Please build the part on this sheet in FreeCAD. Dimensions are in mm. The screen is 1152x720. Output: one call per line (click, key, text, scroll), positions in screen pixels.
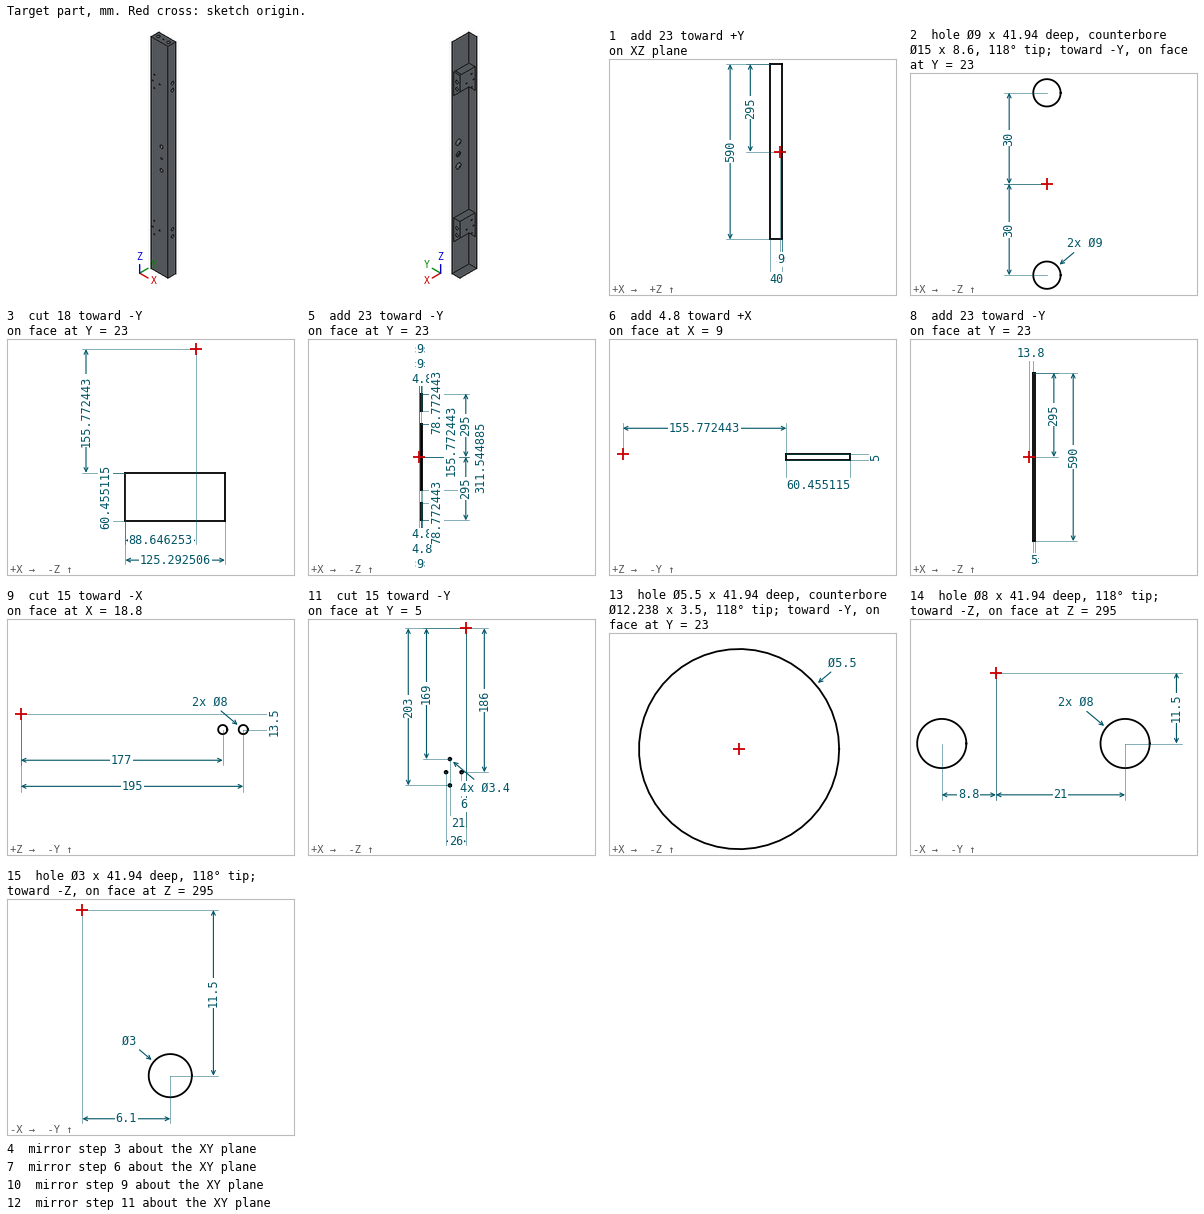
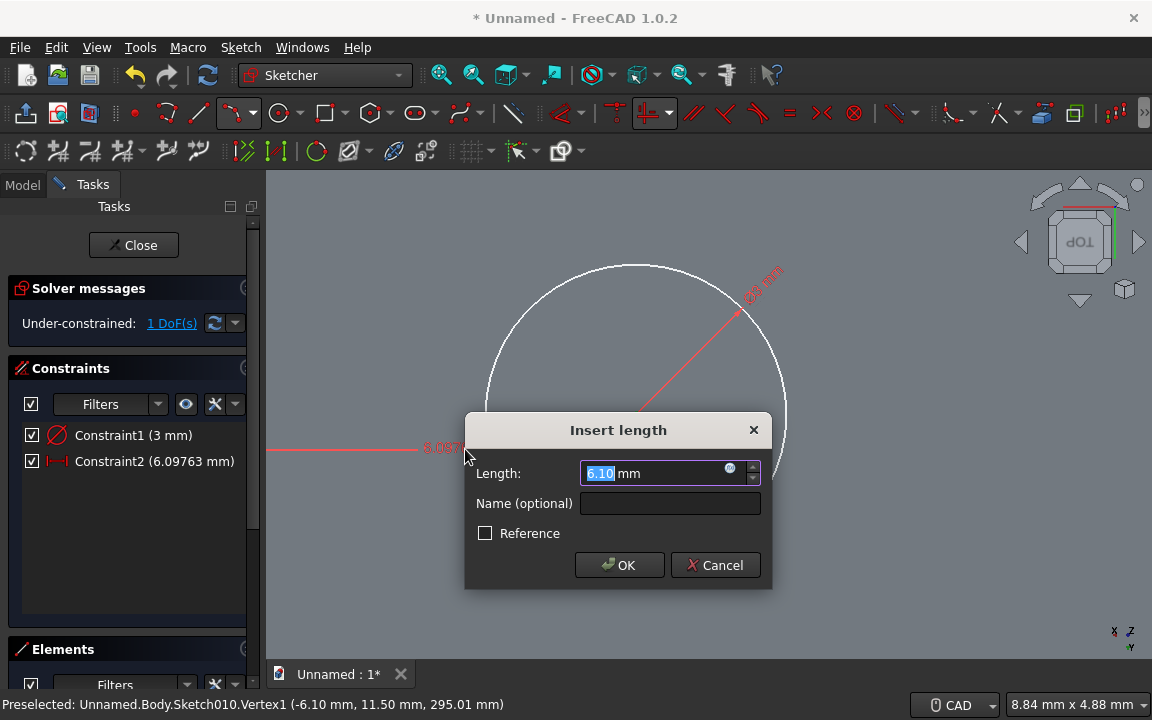
text(6.1)
key(Return)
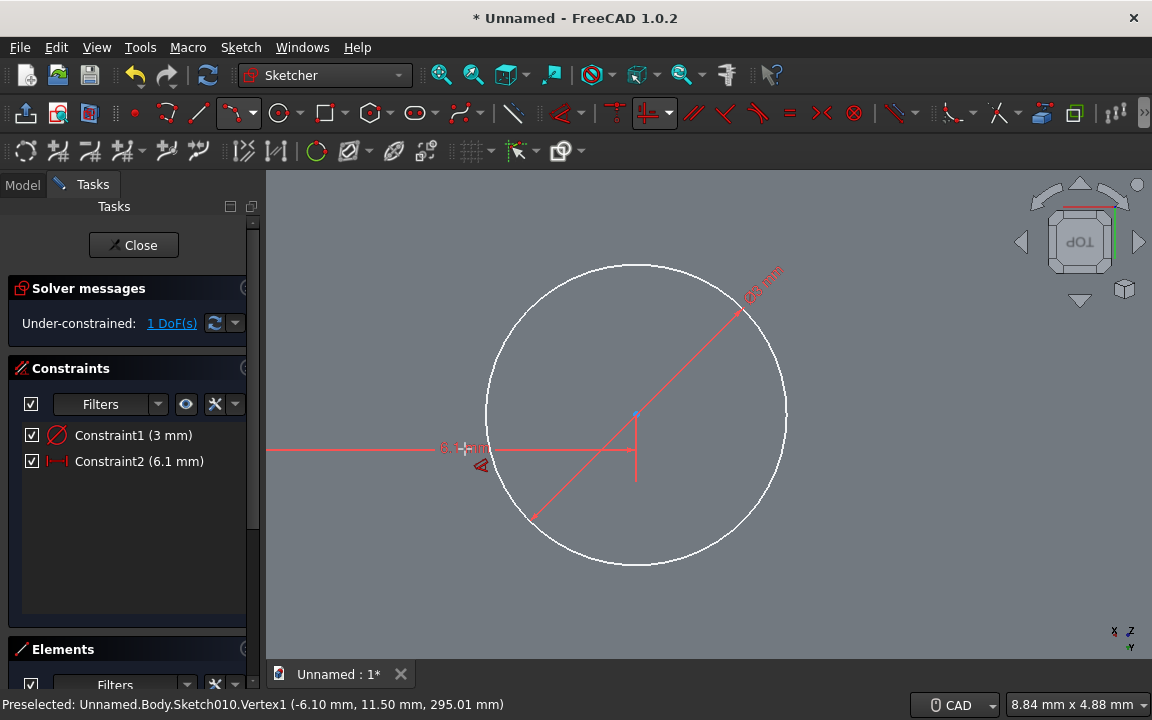
click(636, 415)
click(670, 306)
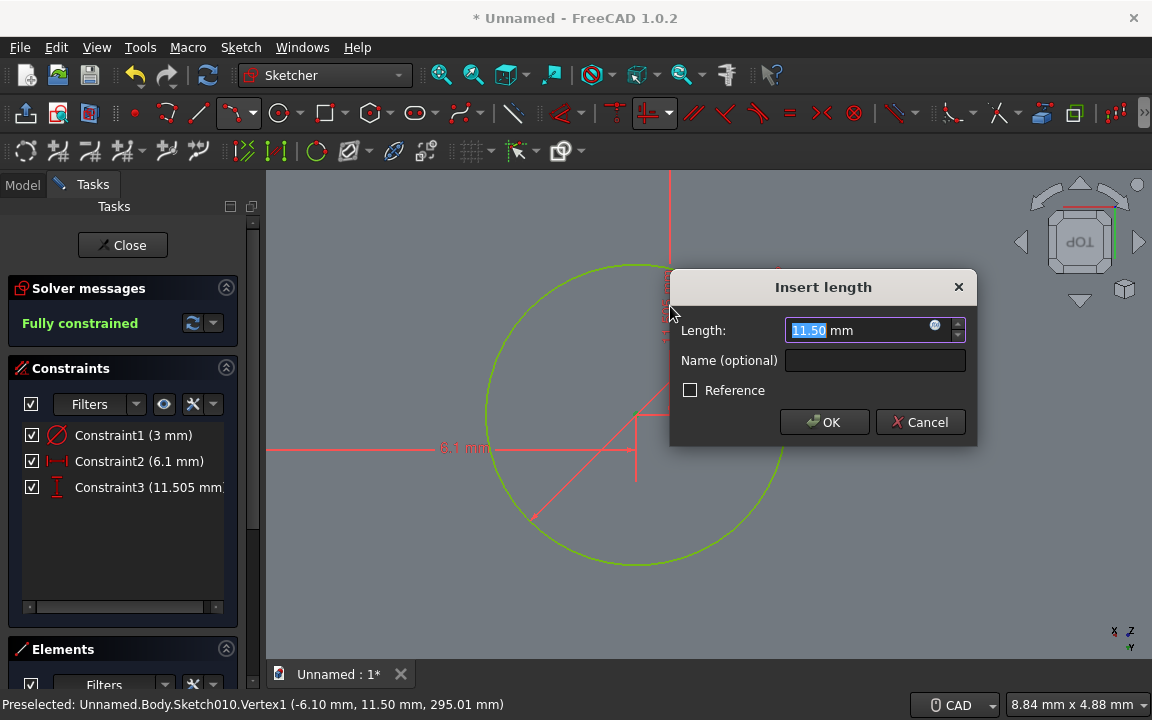
text(11.5)
key(Return)
key(Escape)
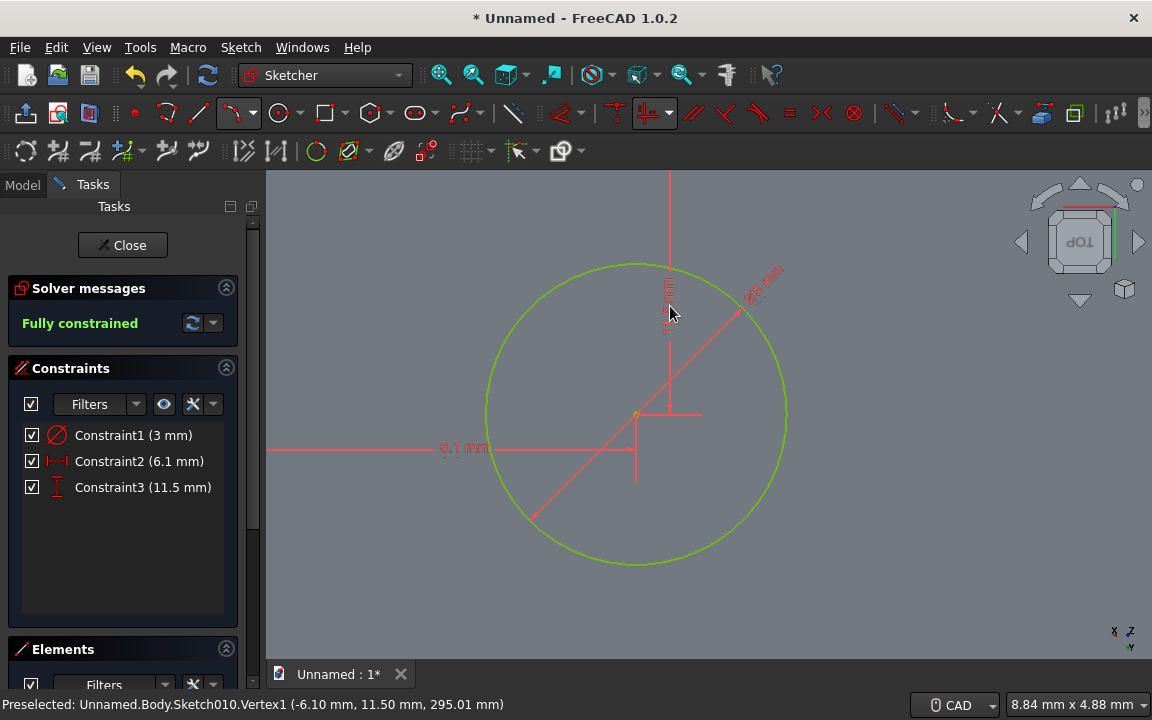
click(123, 245)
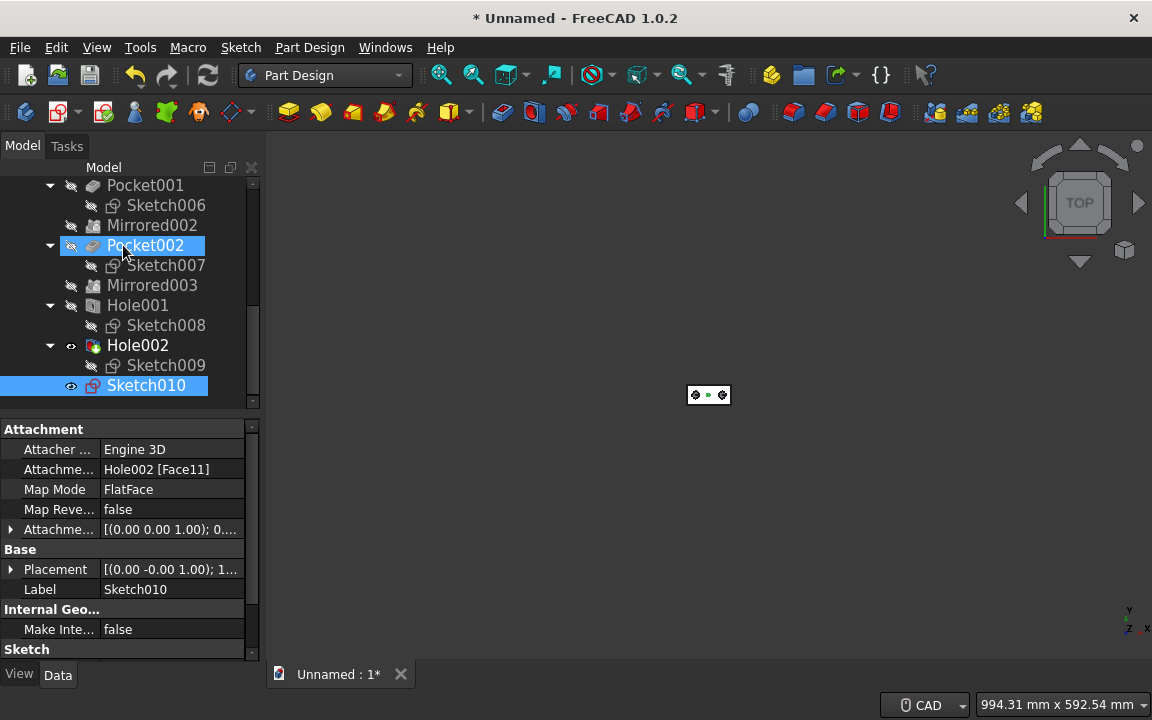
click(536, 112)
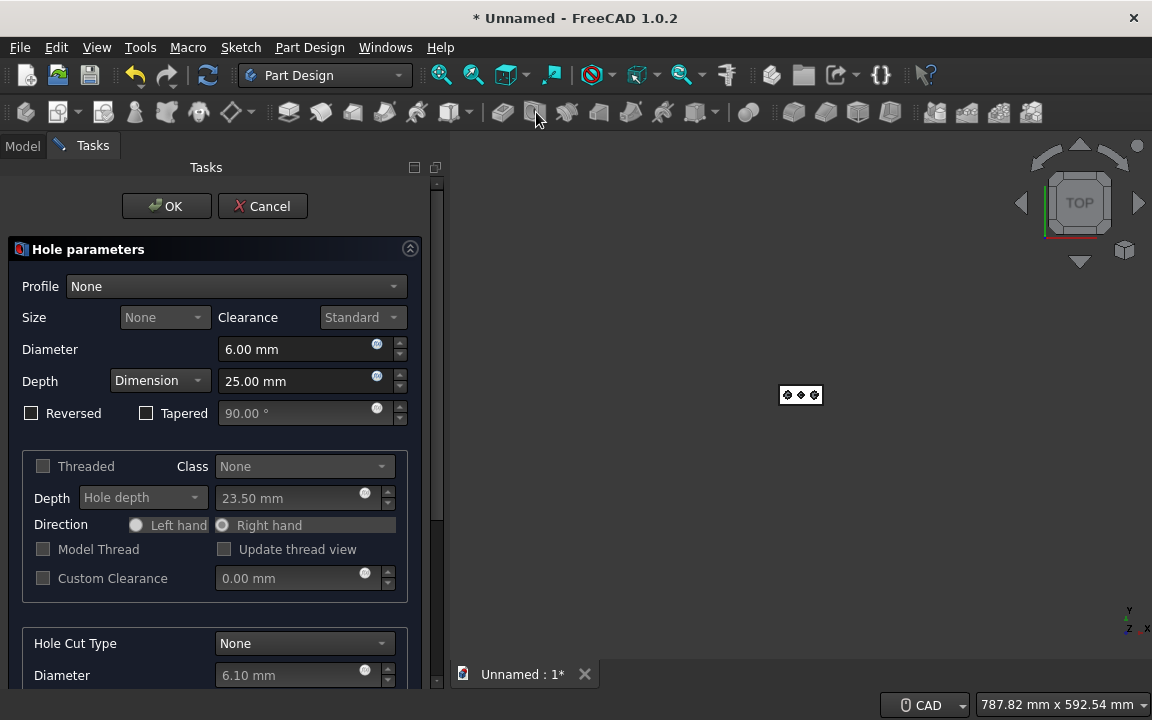
triple_click(305, 349)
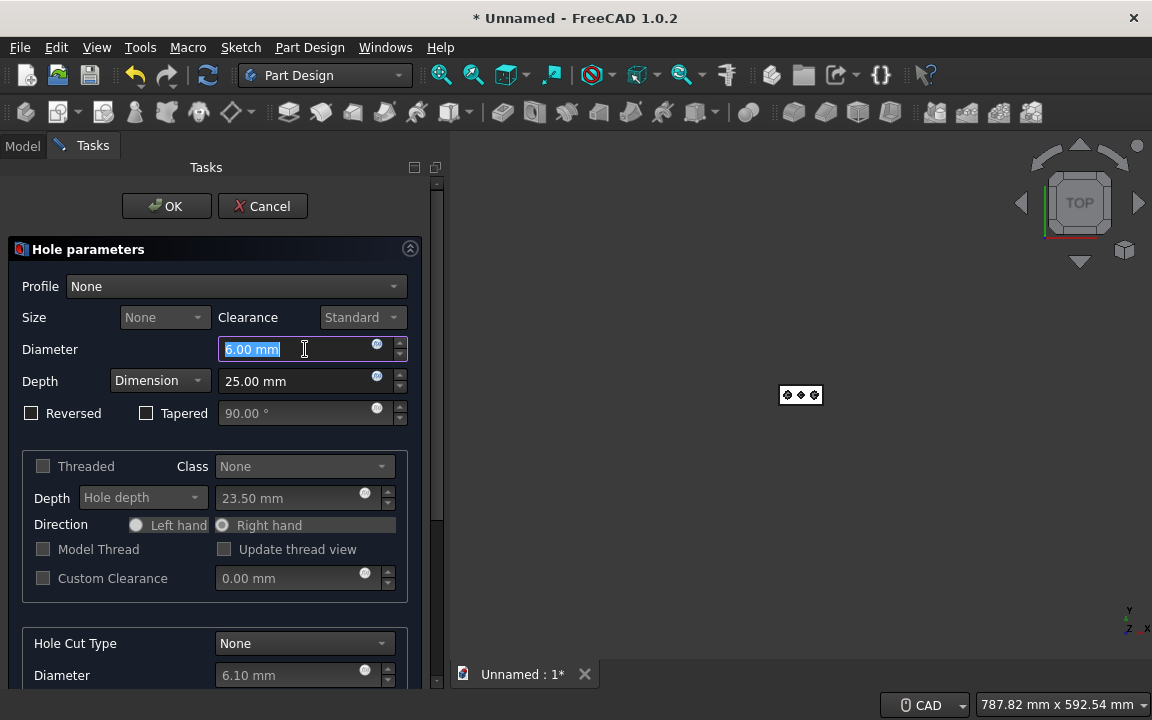
text(3)
key(Tab)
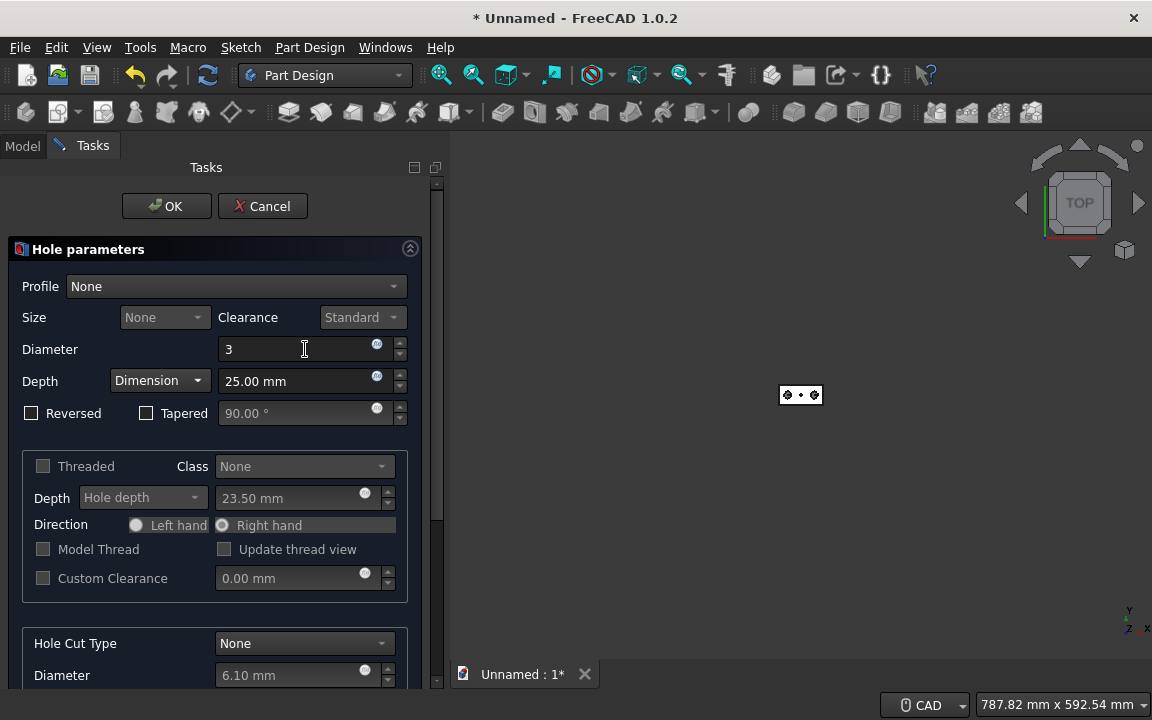
triple_click(305, 381)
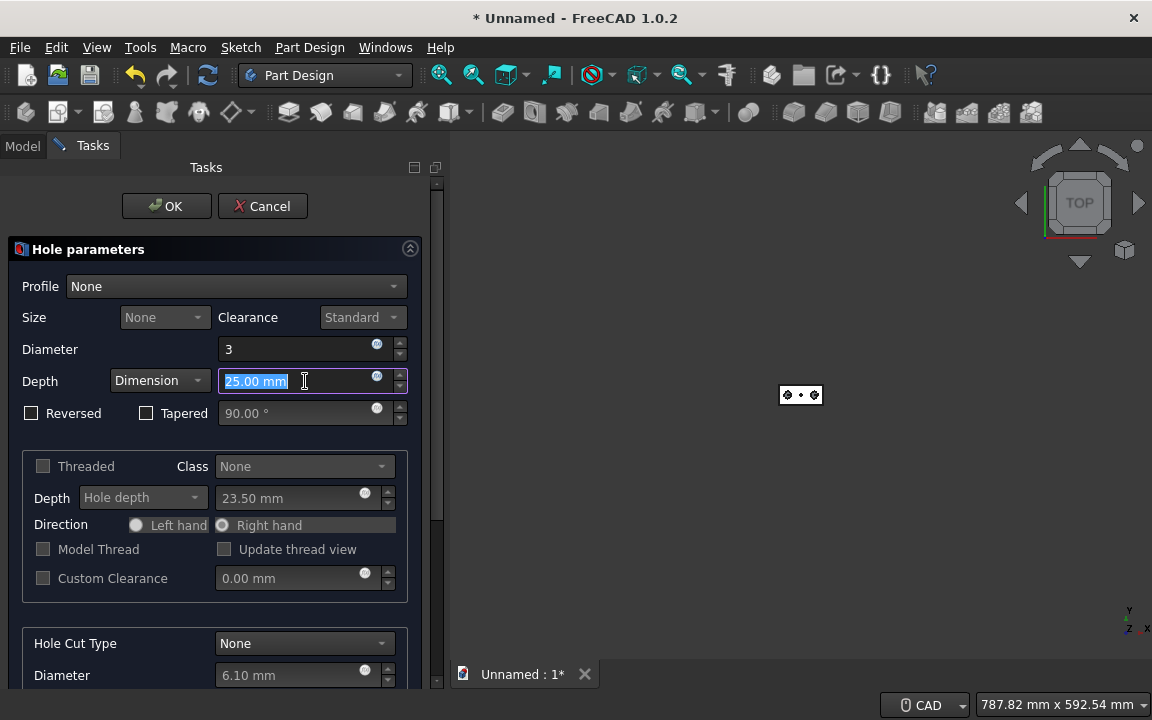
text(41.94)
key(Tab)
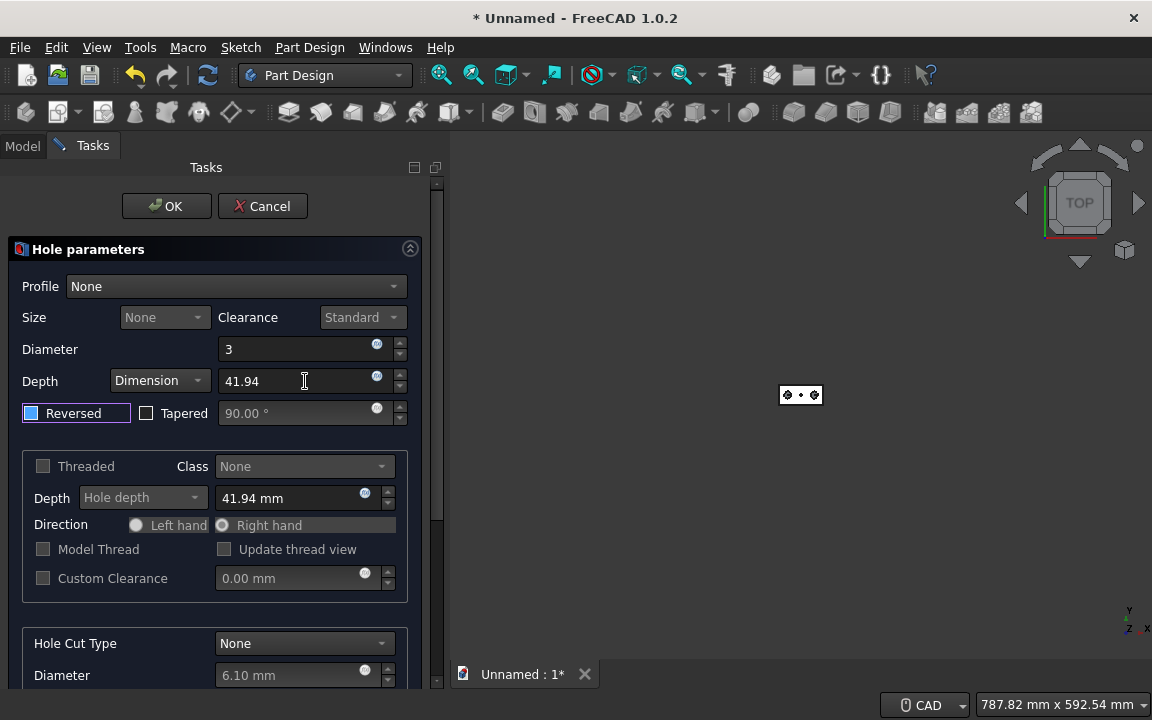
click(167, 206)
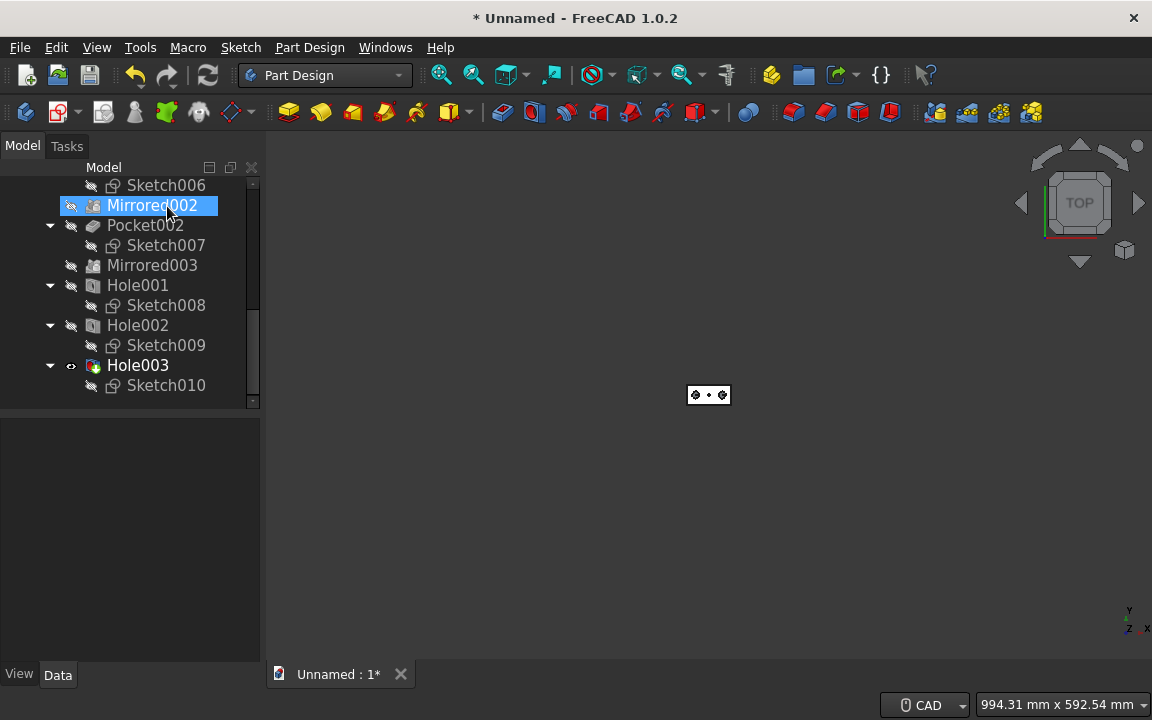
key(0)